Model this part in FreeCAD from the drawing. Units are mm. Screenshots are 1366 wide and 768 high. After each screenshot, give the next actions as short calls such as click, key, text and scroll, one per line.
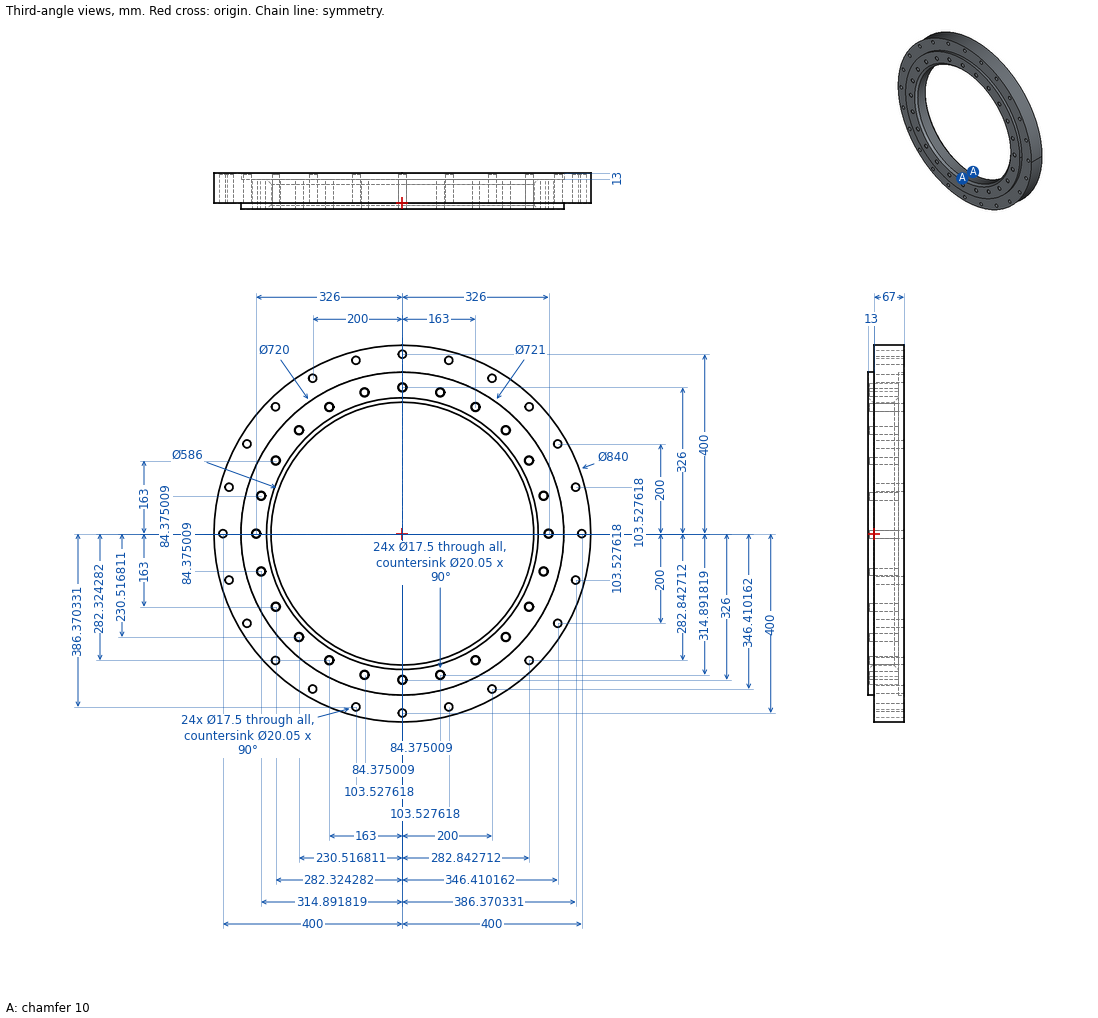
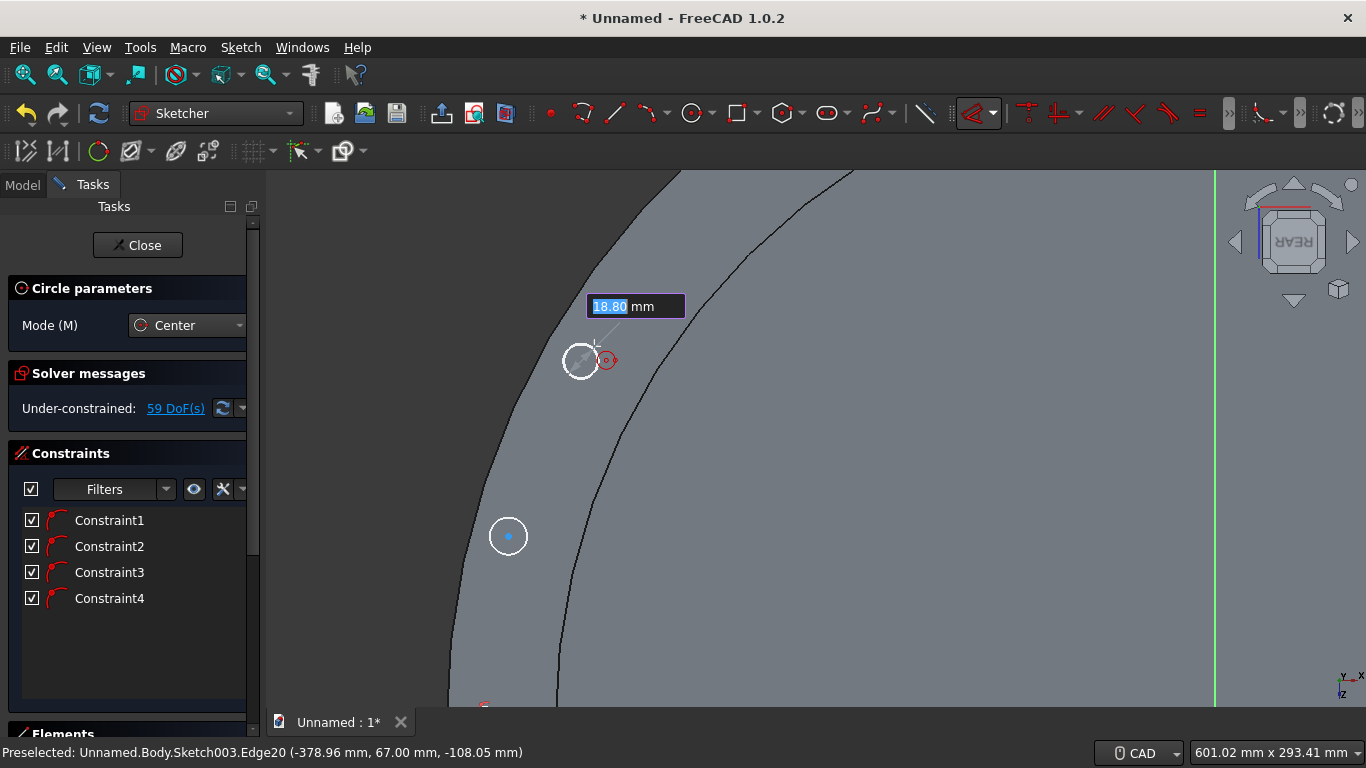
click(593, 344)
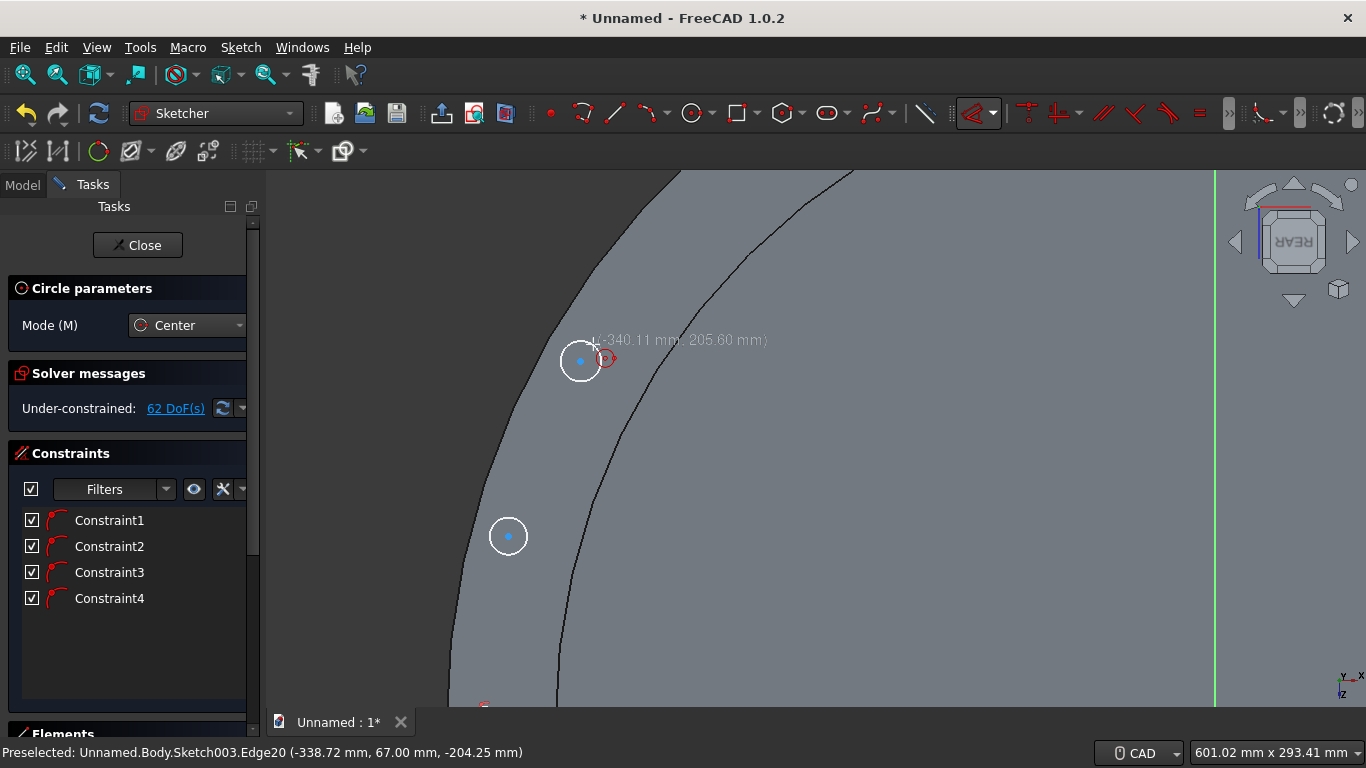
scroll(698, 204, up, 2)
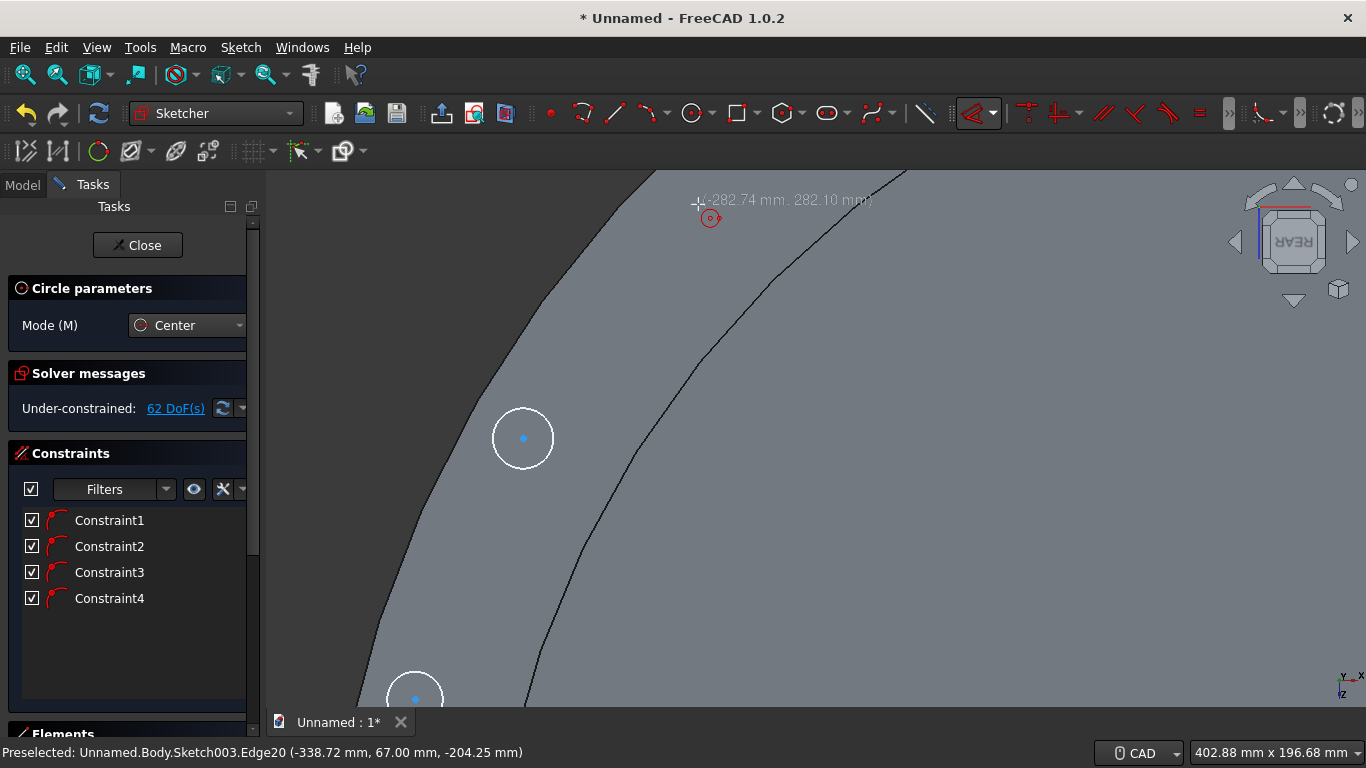
scroll(604, 332, down, 9)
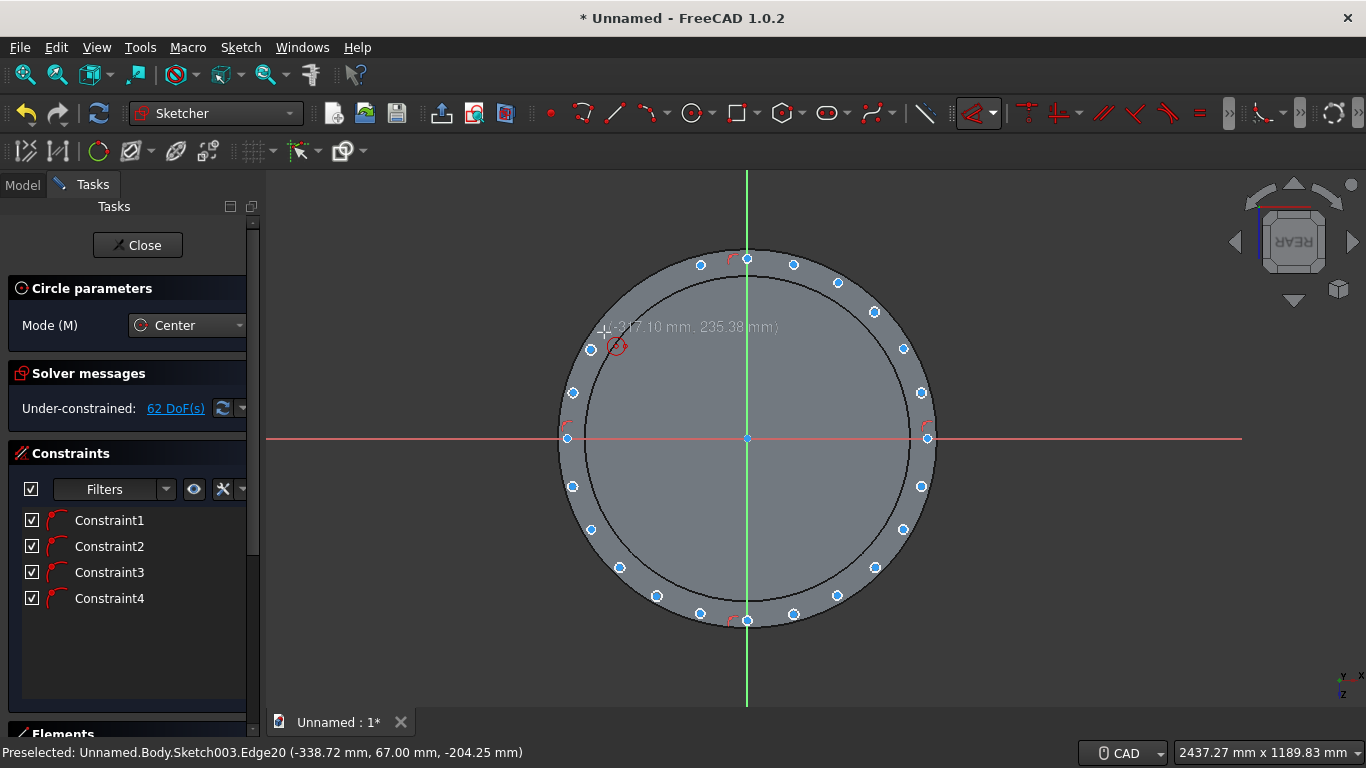
click(620, 311)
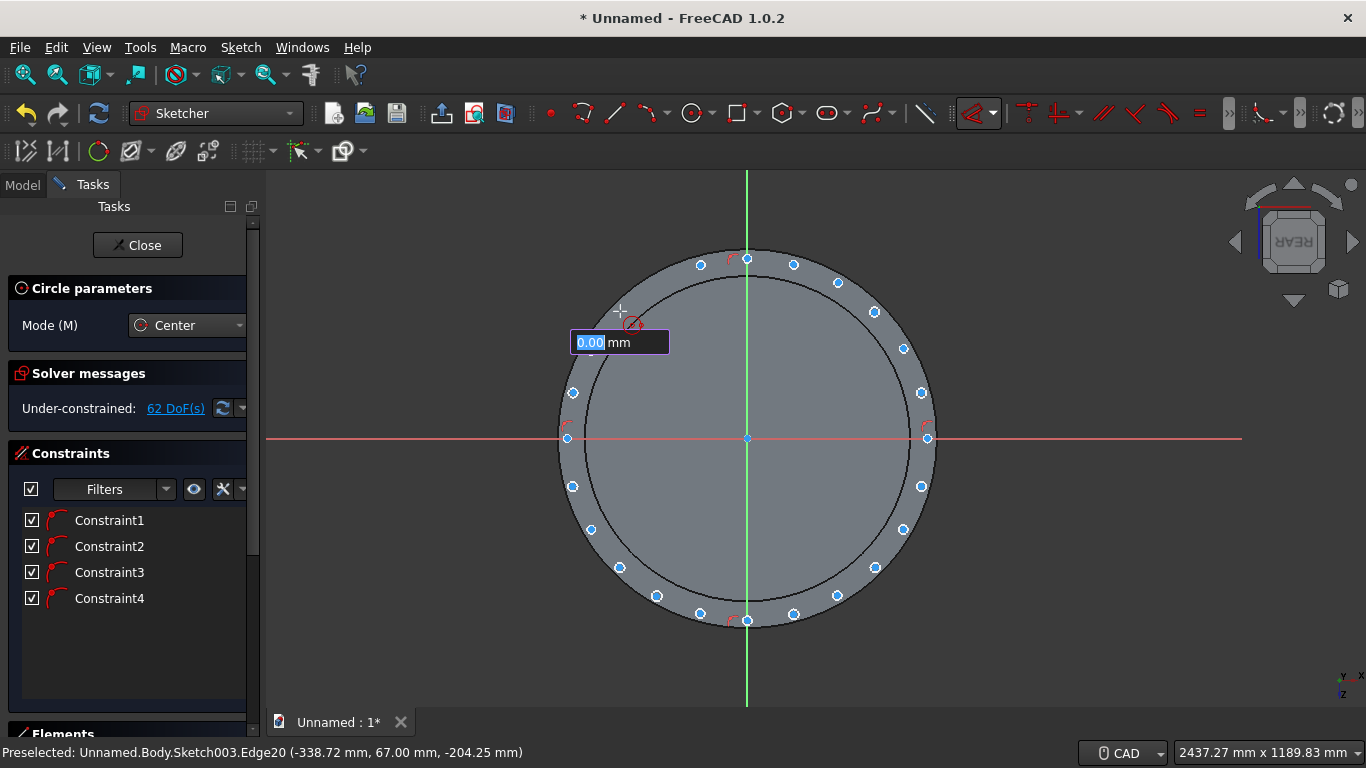
scroll(623, 308, up, 7)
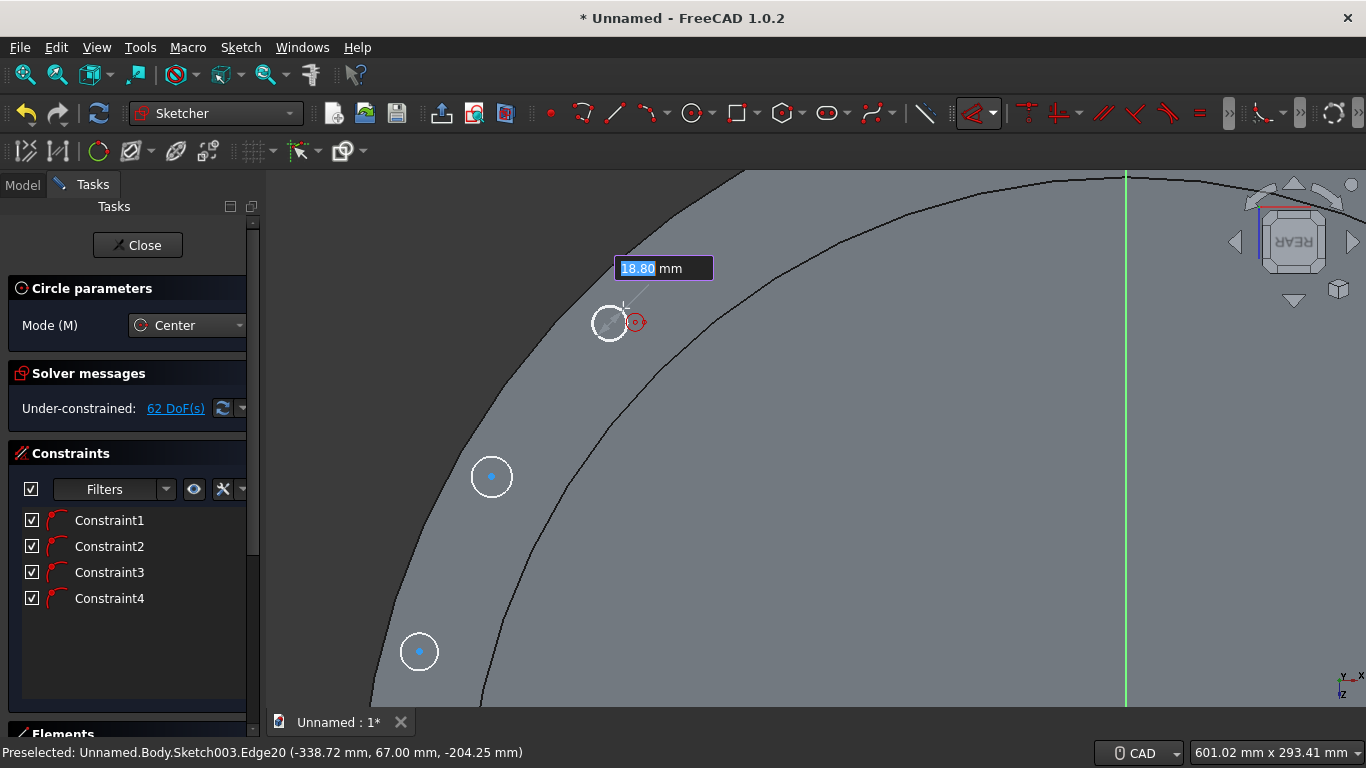
click(620, 308)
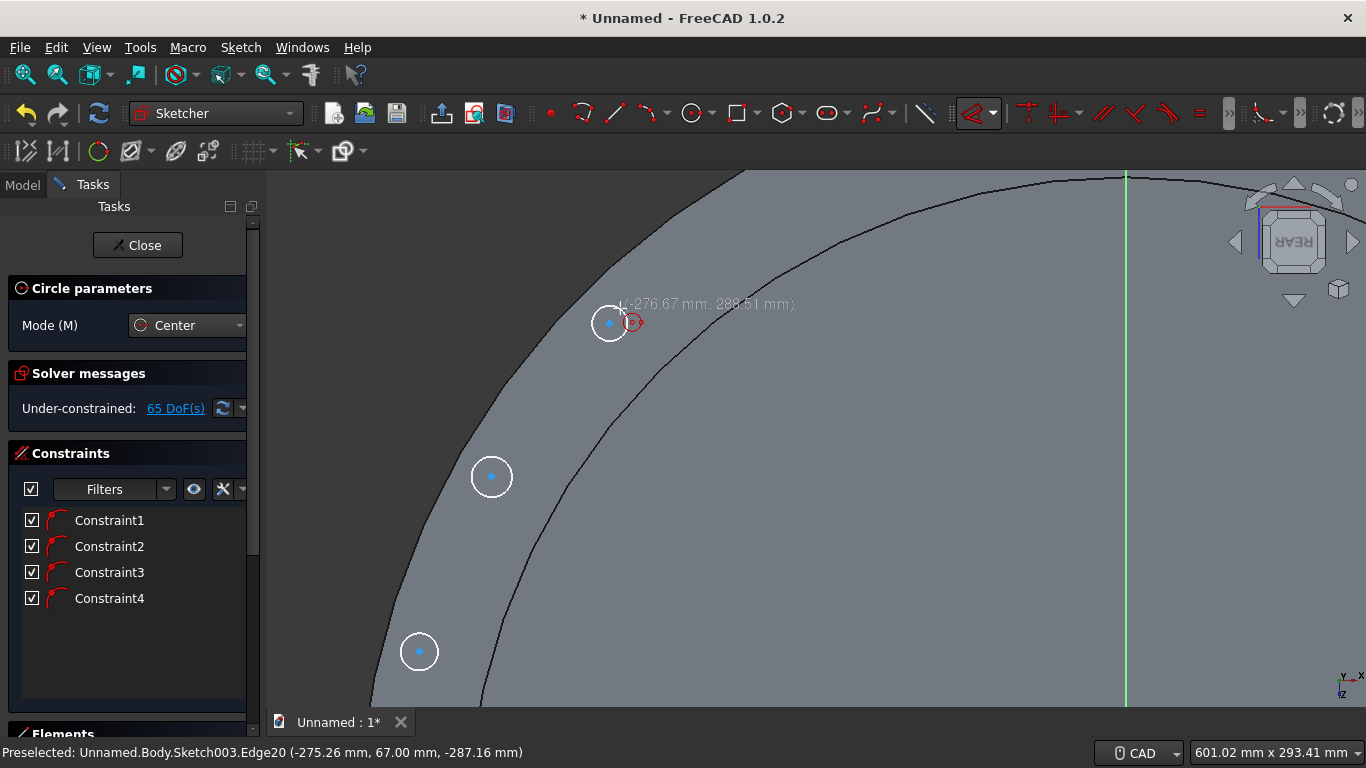
scroll(760, 203, up, 2)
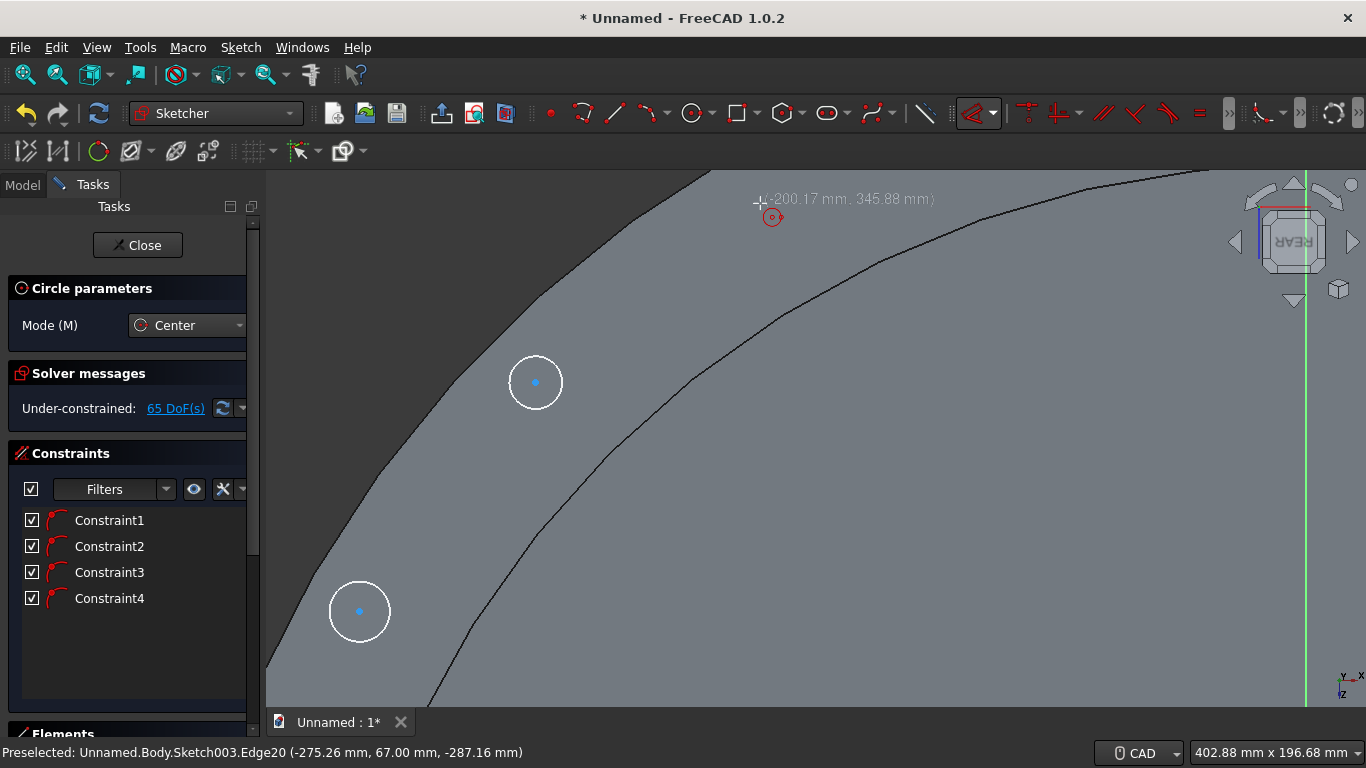
scroll(637, 298, down, 9)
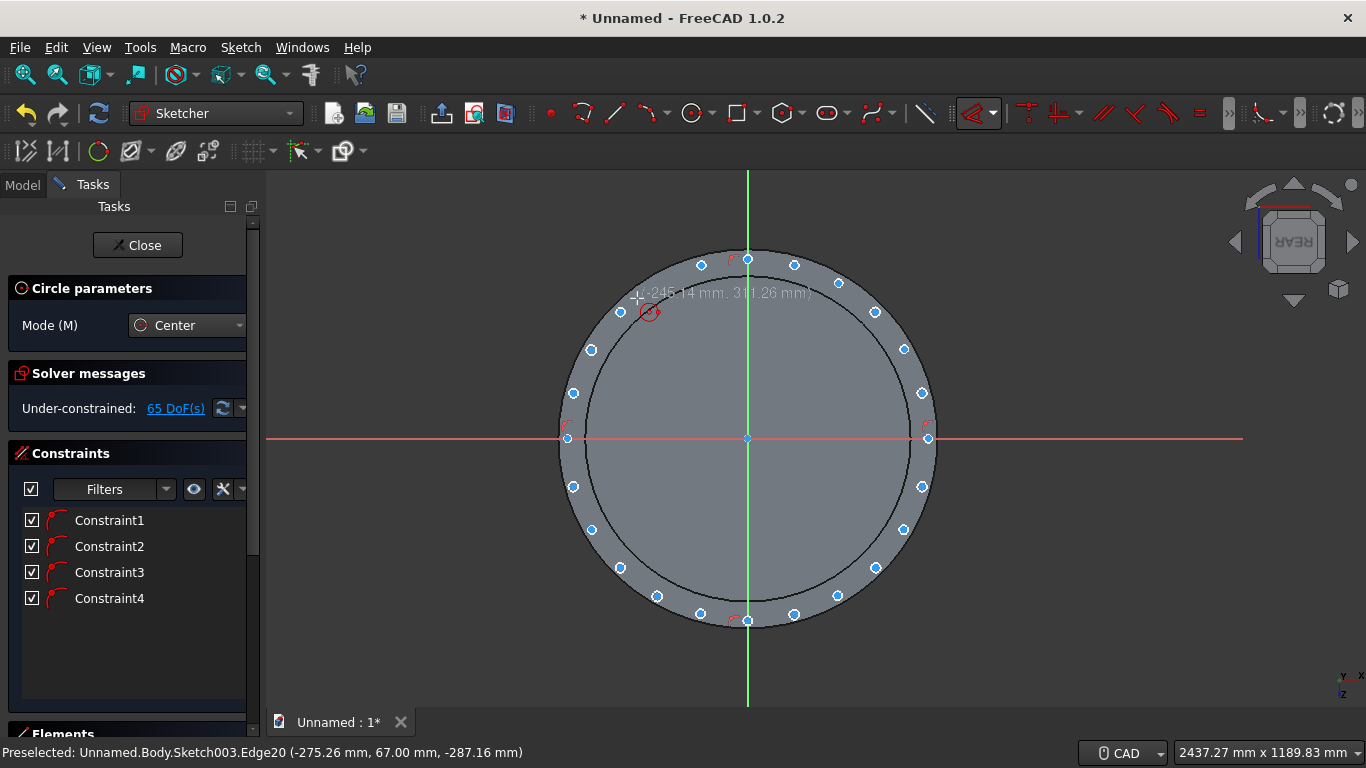
click(658, 282)